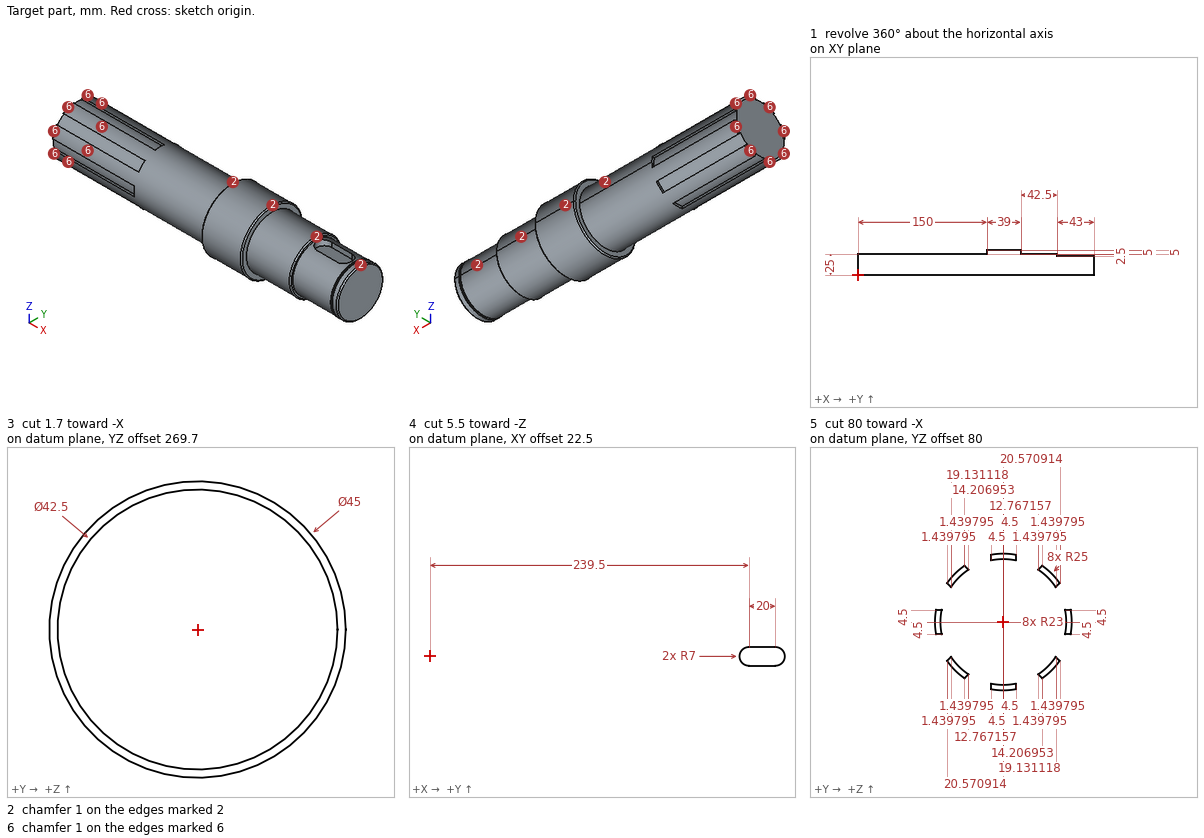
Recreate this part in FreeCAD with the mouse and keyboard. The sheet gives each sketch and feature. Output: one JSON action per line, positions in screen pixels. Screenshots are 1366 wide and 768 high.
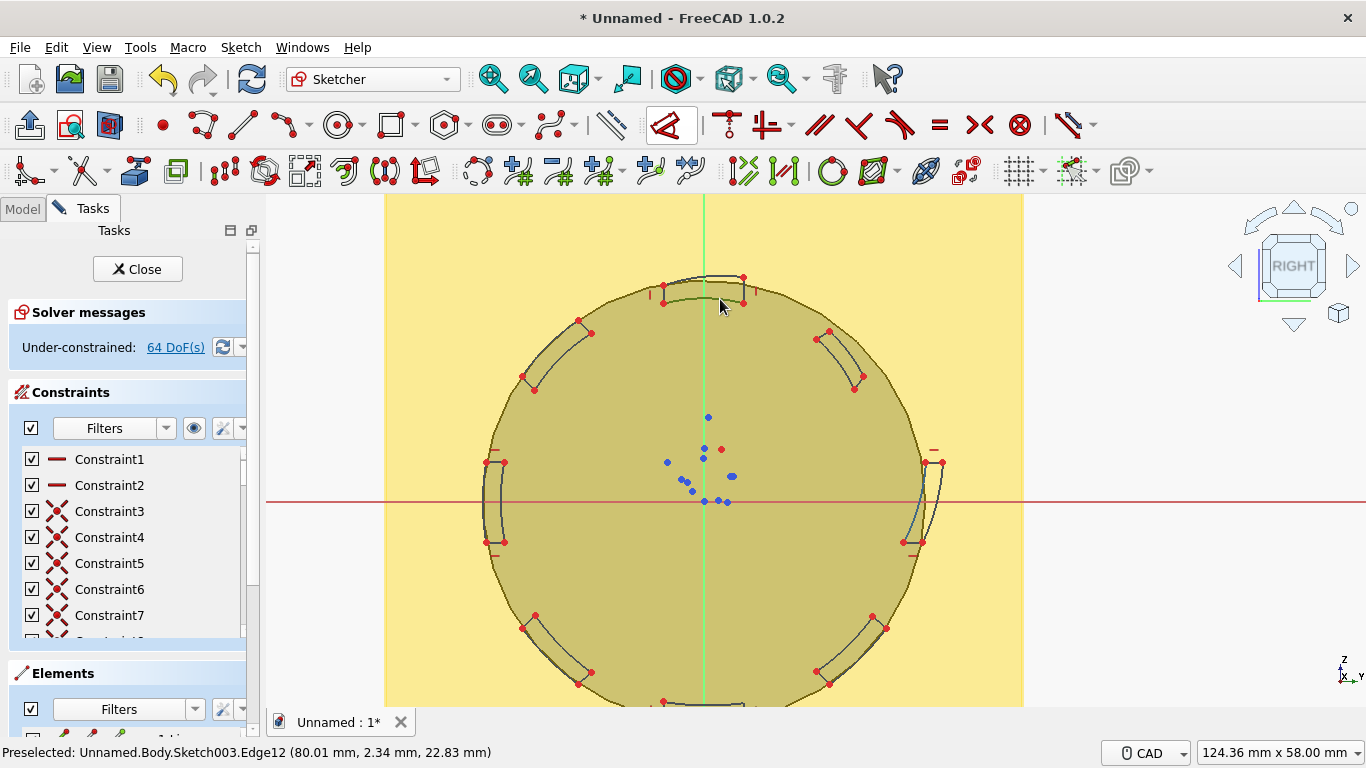
{"action": "left_click", "coordinate": [728, 126]}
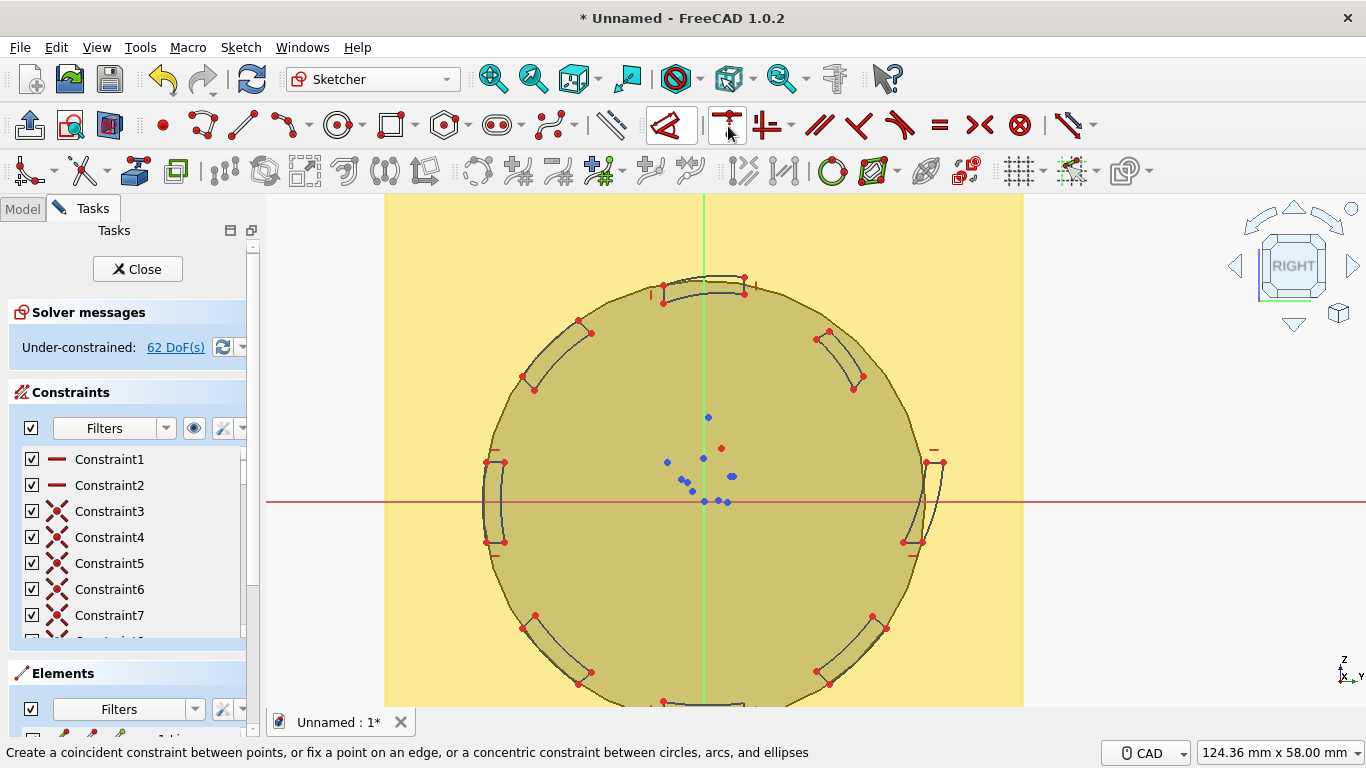
{"action": "left_click", "coordinate": [914, 520]}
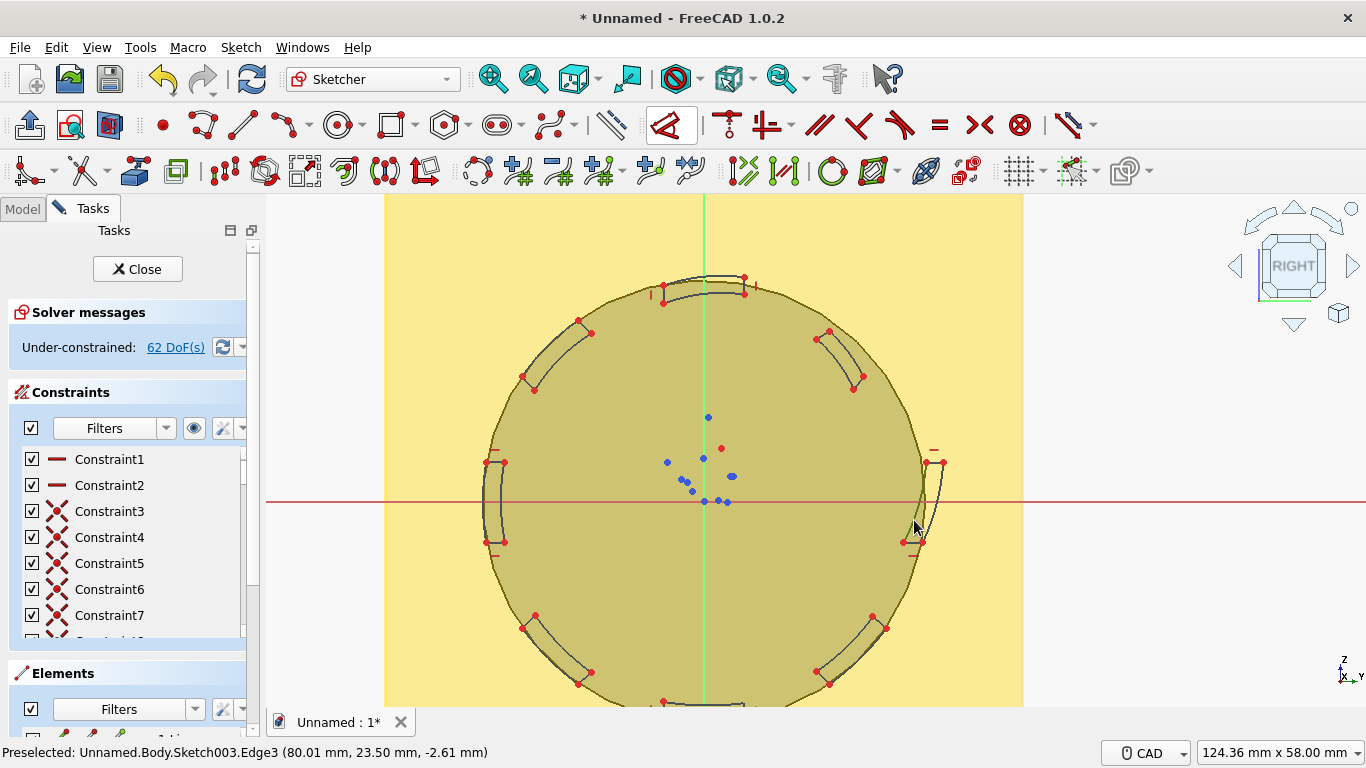
{"action": "left_click", "coordinate": [559, 335]}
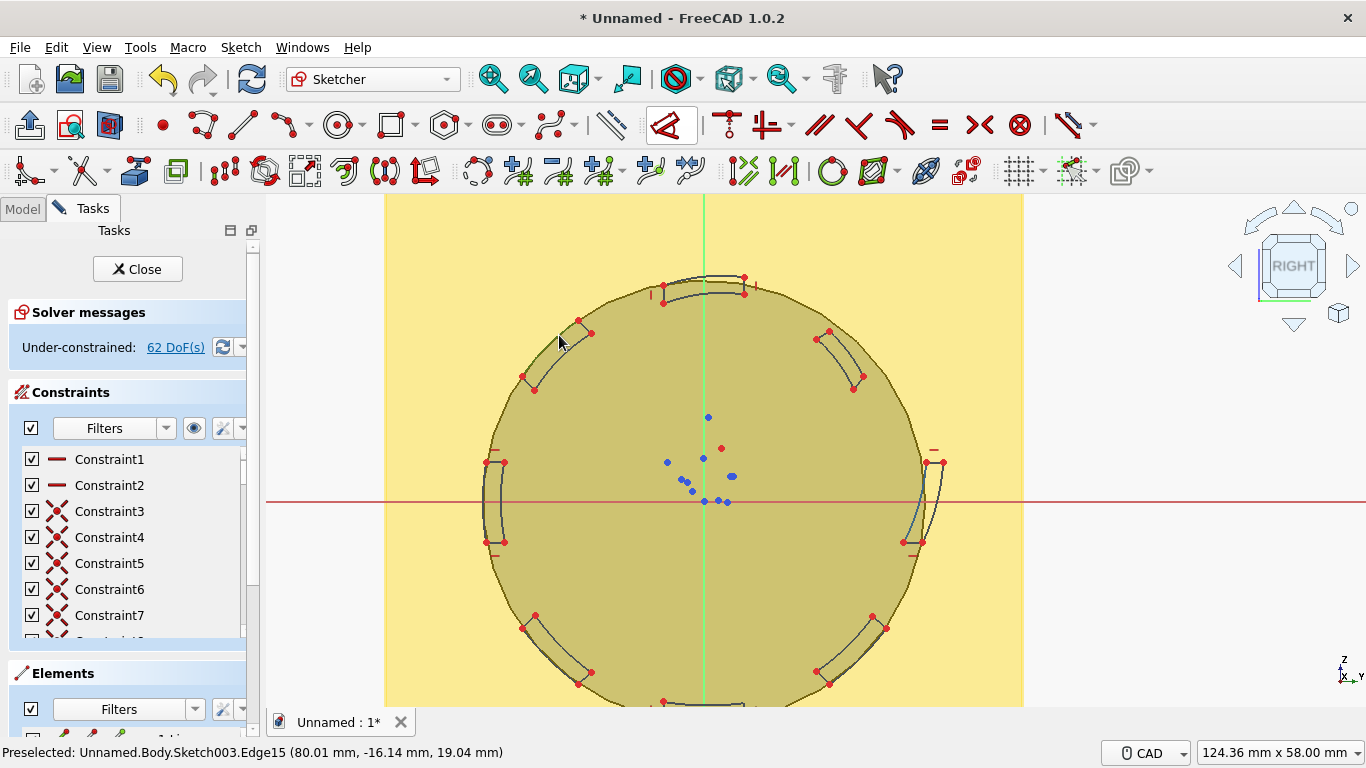
{"action": "left_click", "coordinate": [728, 126]}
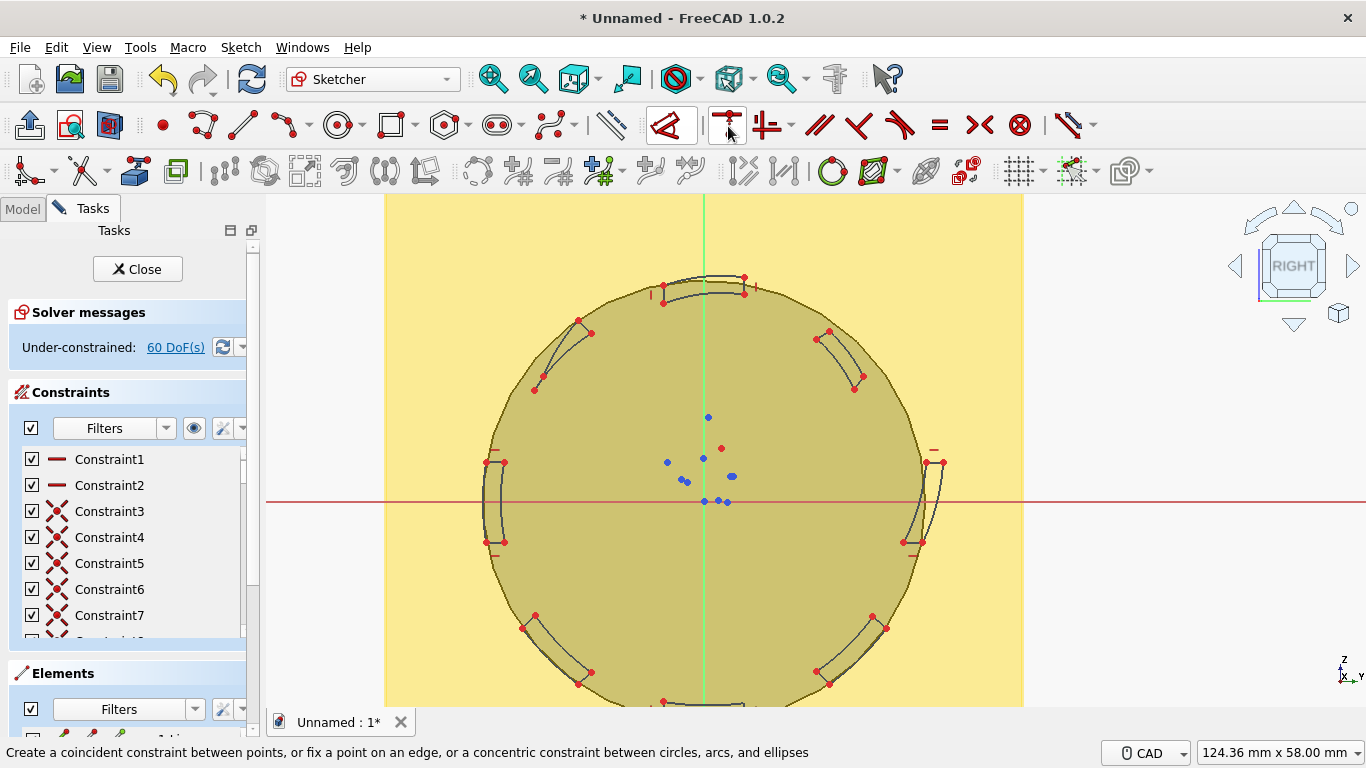
{"action": "left_click", "coordinate": [914, 520]}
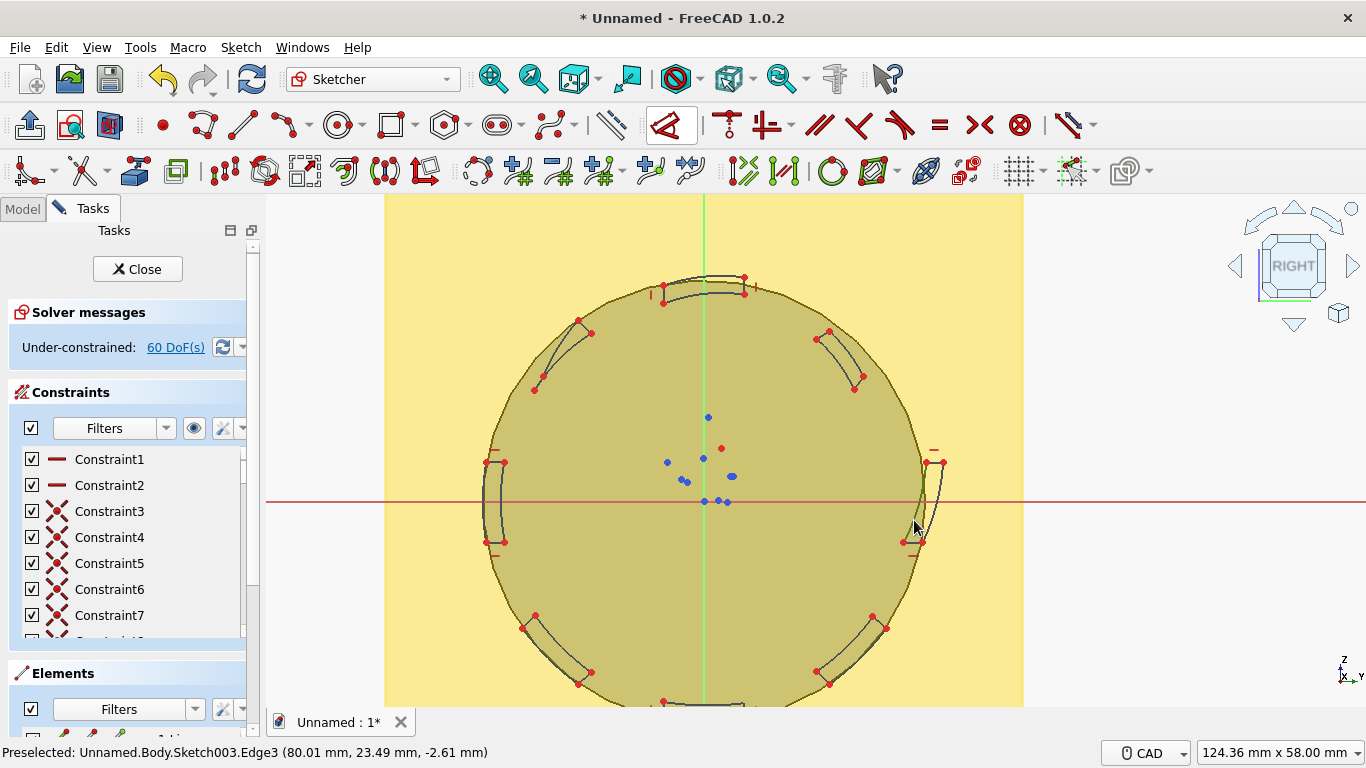
{"action": "left_click", "coordinate": [571, 348]}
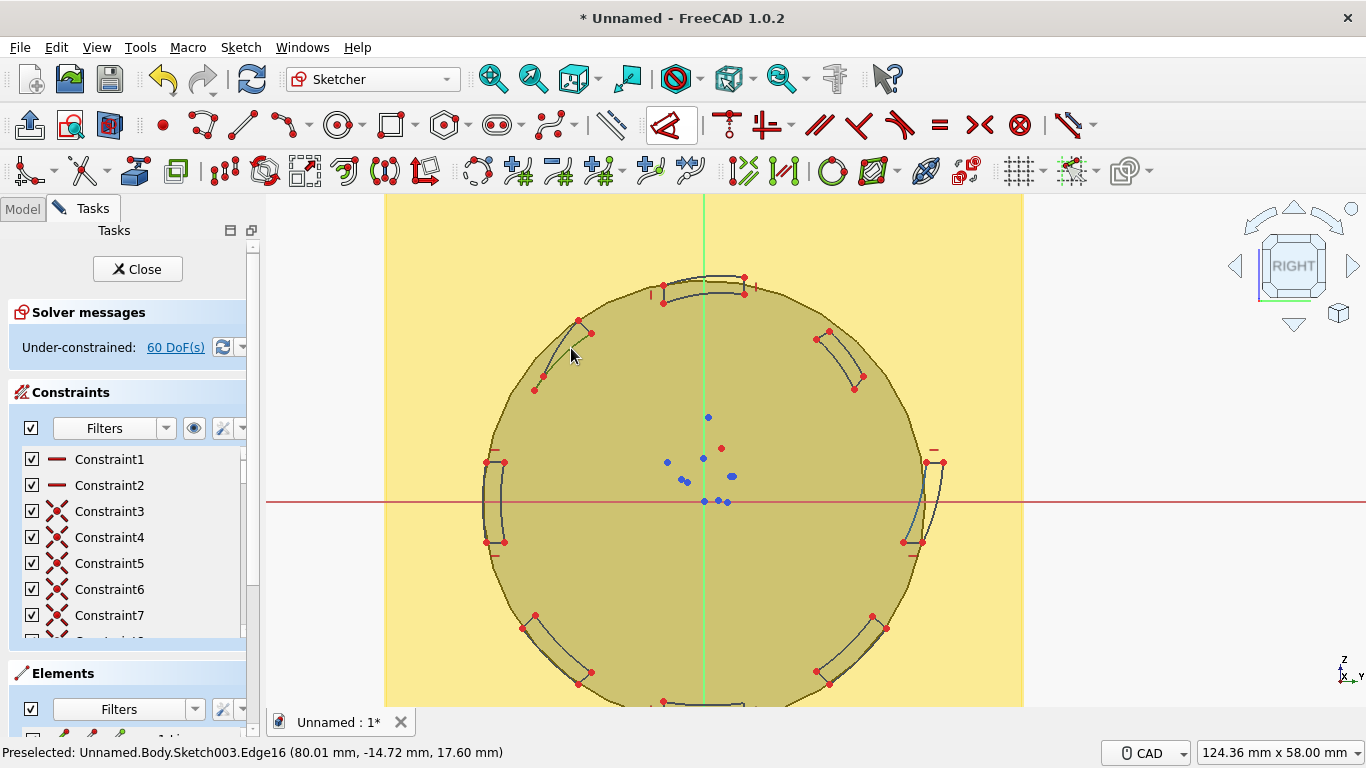
{"action": "left_click", "coordinate": [728, 126]}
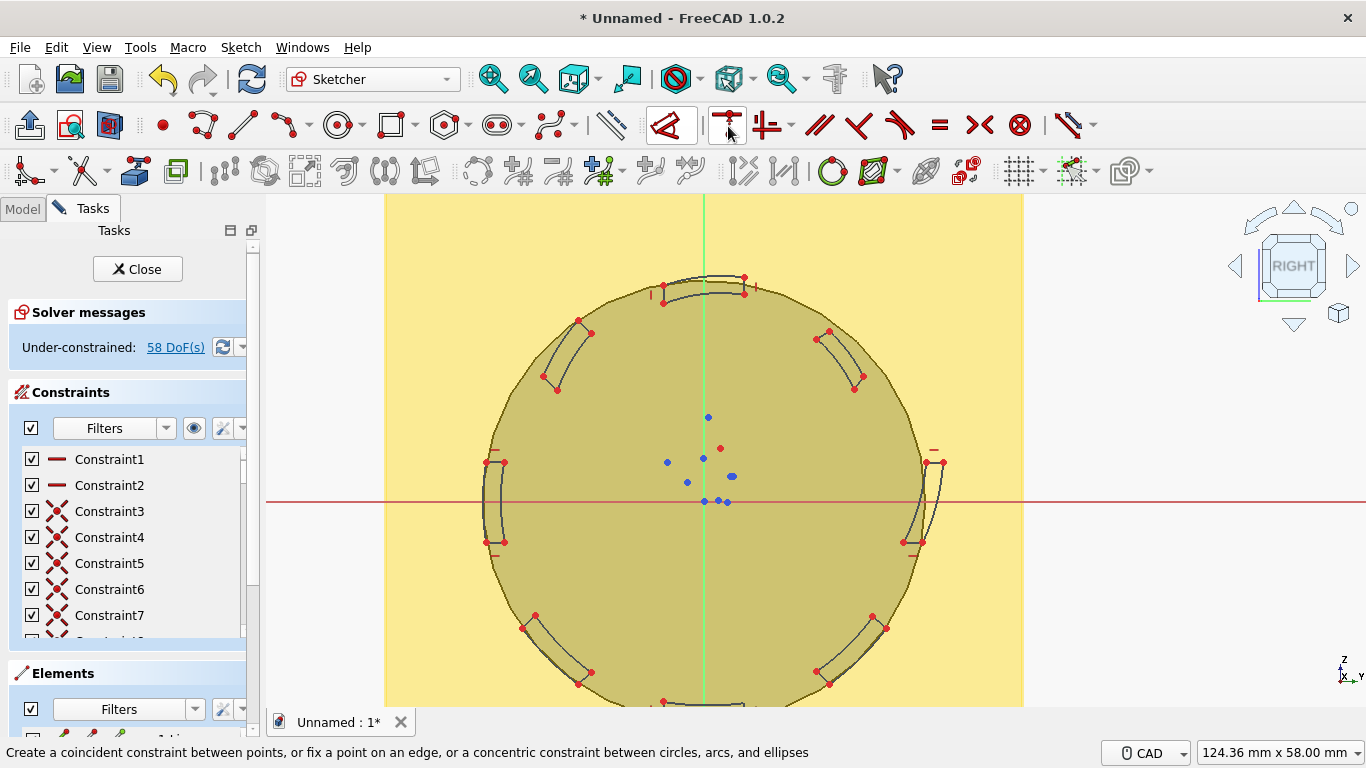
{"action": "left_click", "coordinate": [914, 520]}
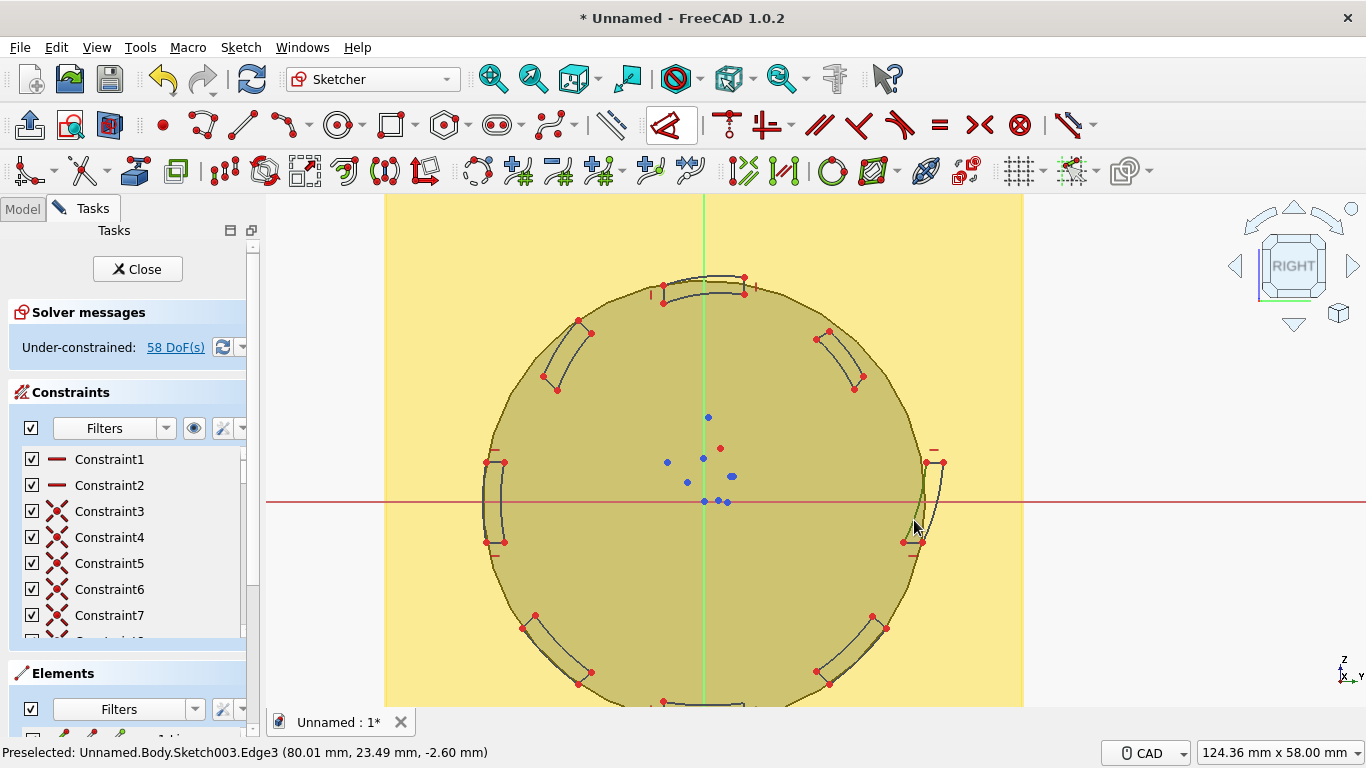
{"action": "left_click", "coordinate": [483, 486]}